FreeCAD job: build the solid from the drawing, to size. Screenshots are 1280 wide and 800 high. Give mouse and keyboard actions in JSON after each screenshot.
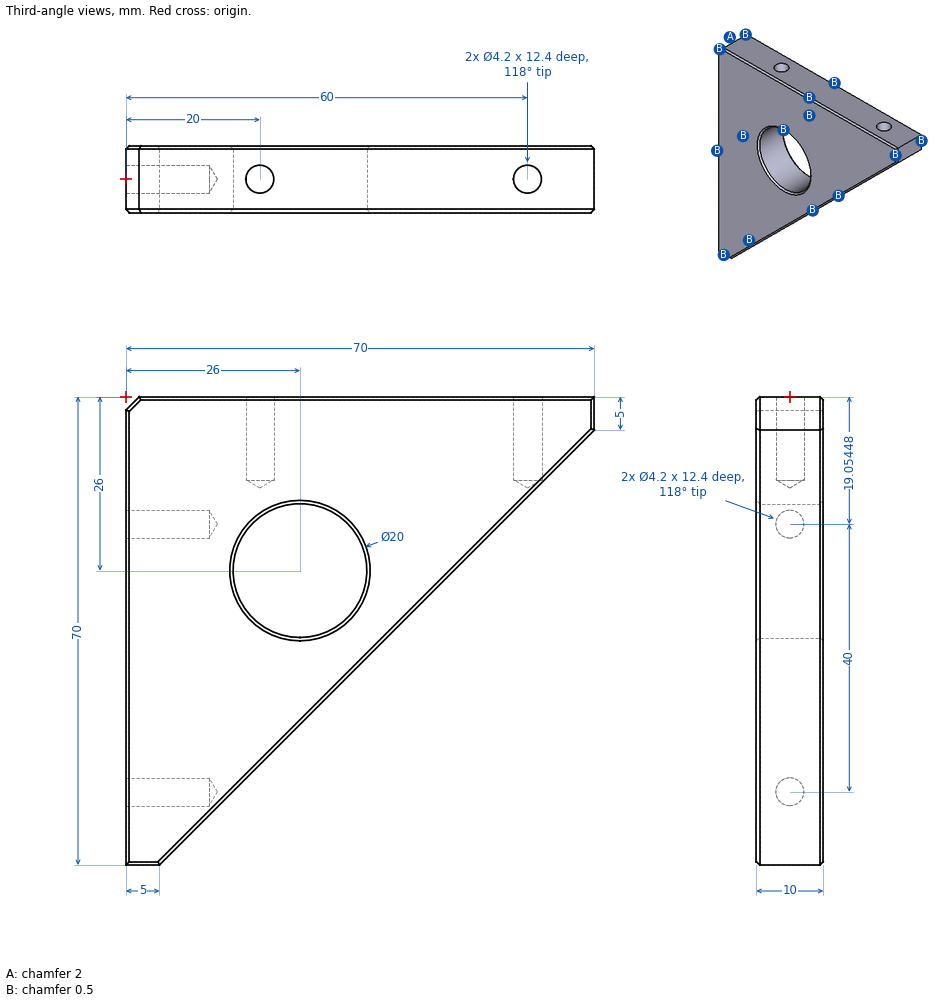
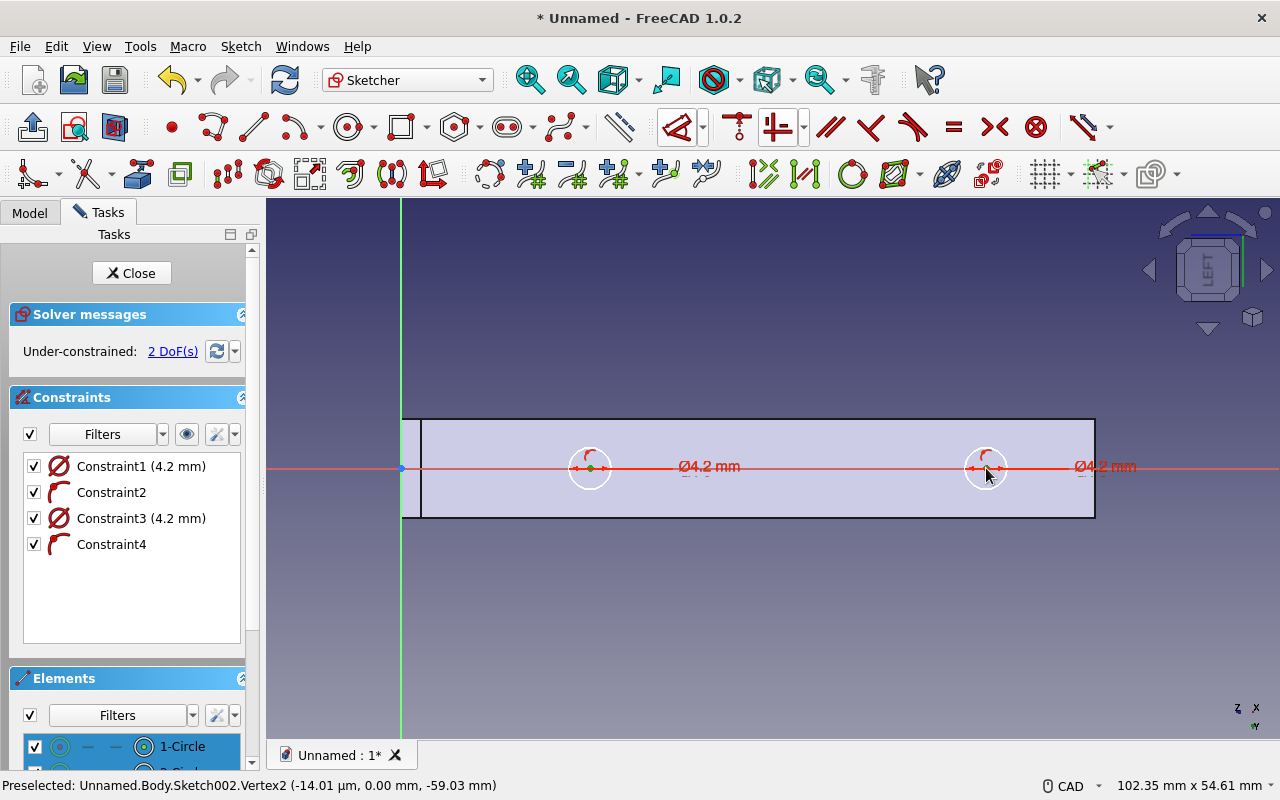
{"action": "key", "text": "l"}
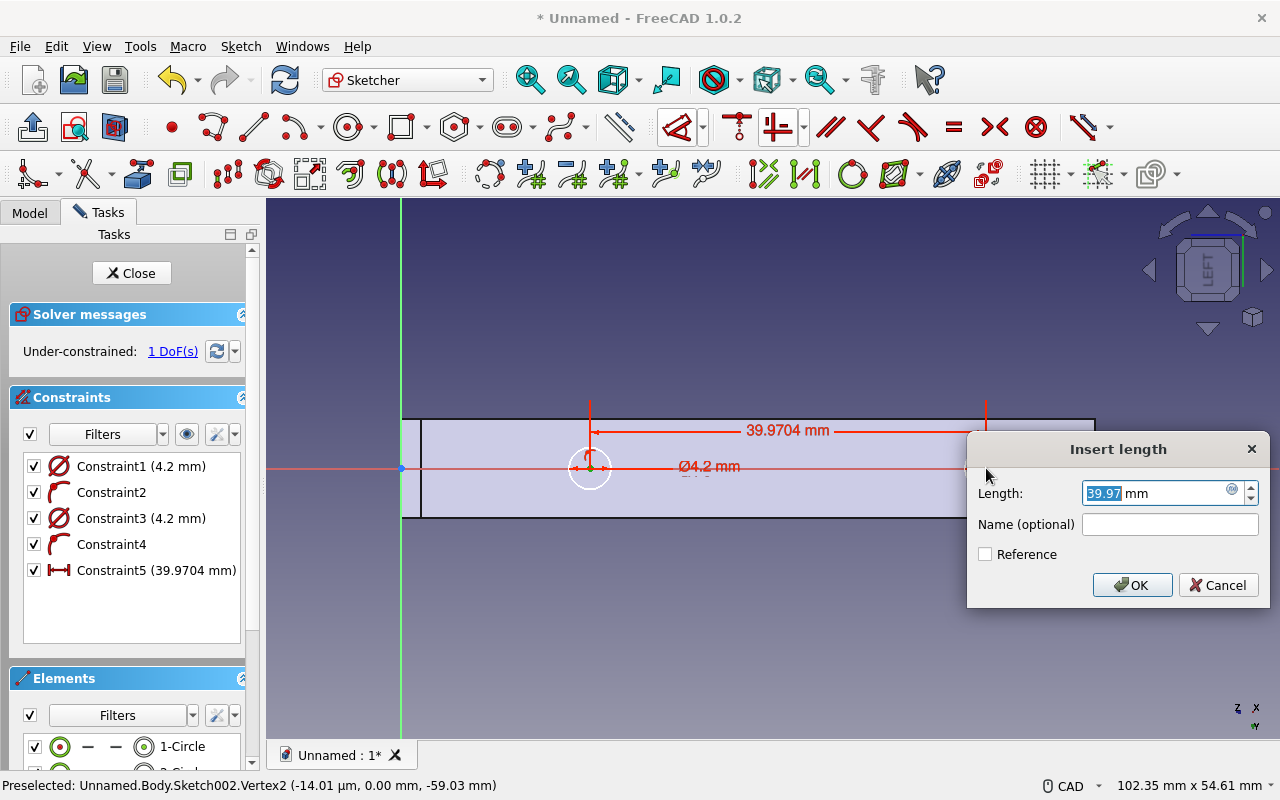
{"action": "type", "text": "40"}
{"action": "key", "text": "Return"}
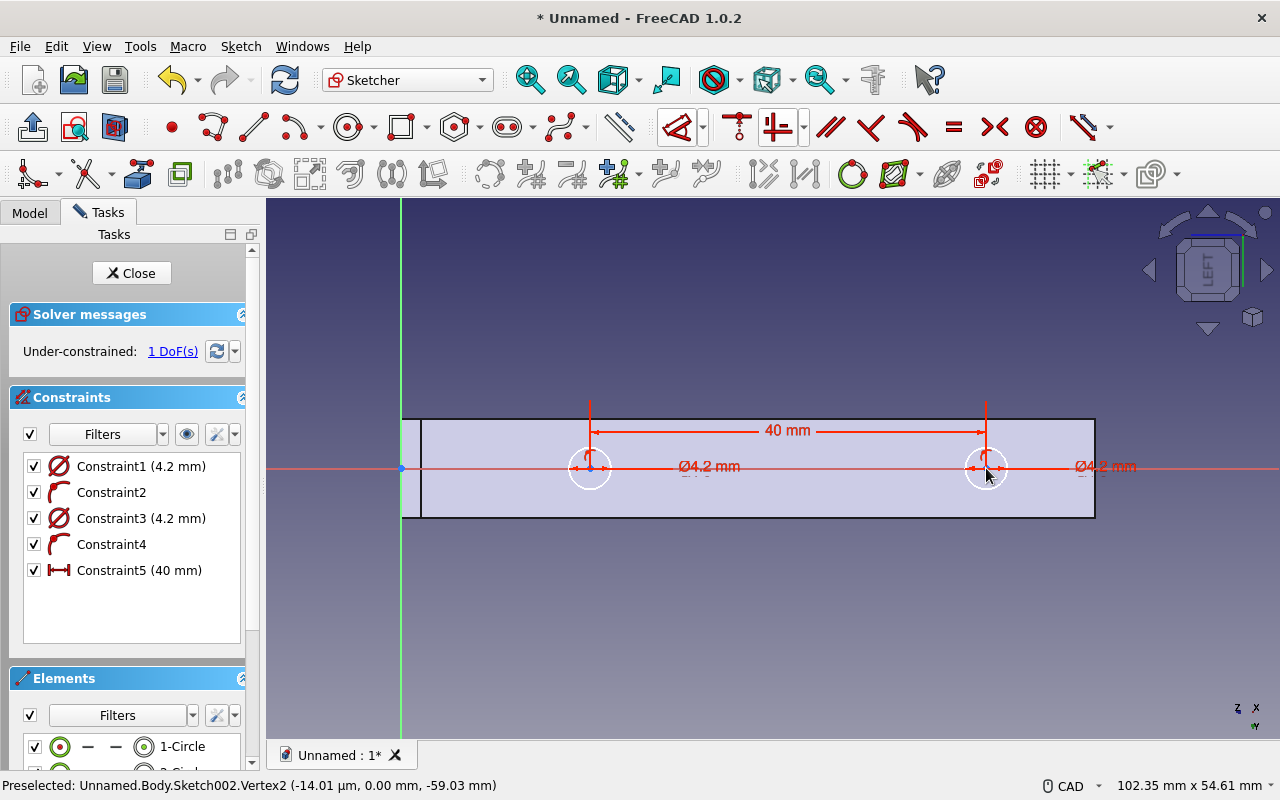
{"action": "left_click", "coordinate": [590, 468]}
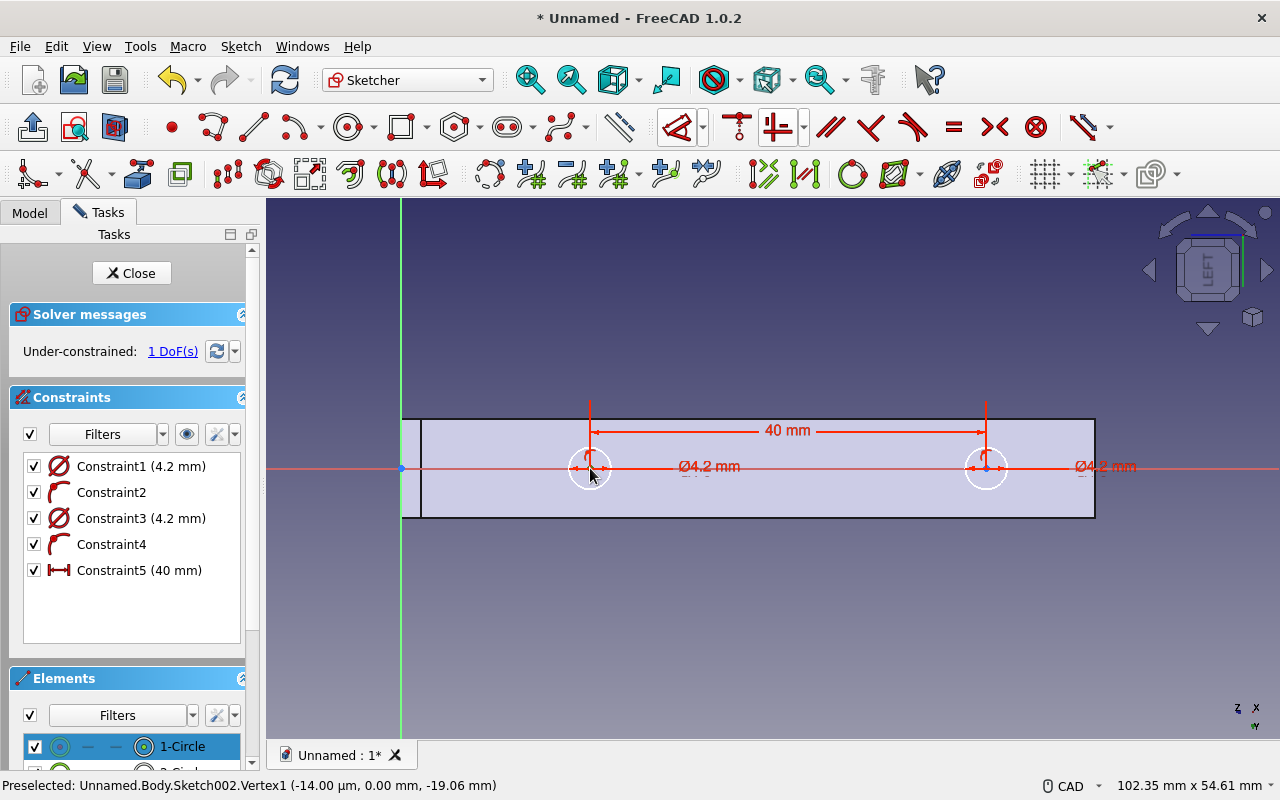
{"action": "left_click", "coordinate": [702, 128]}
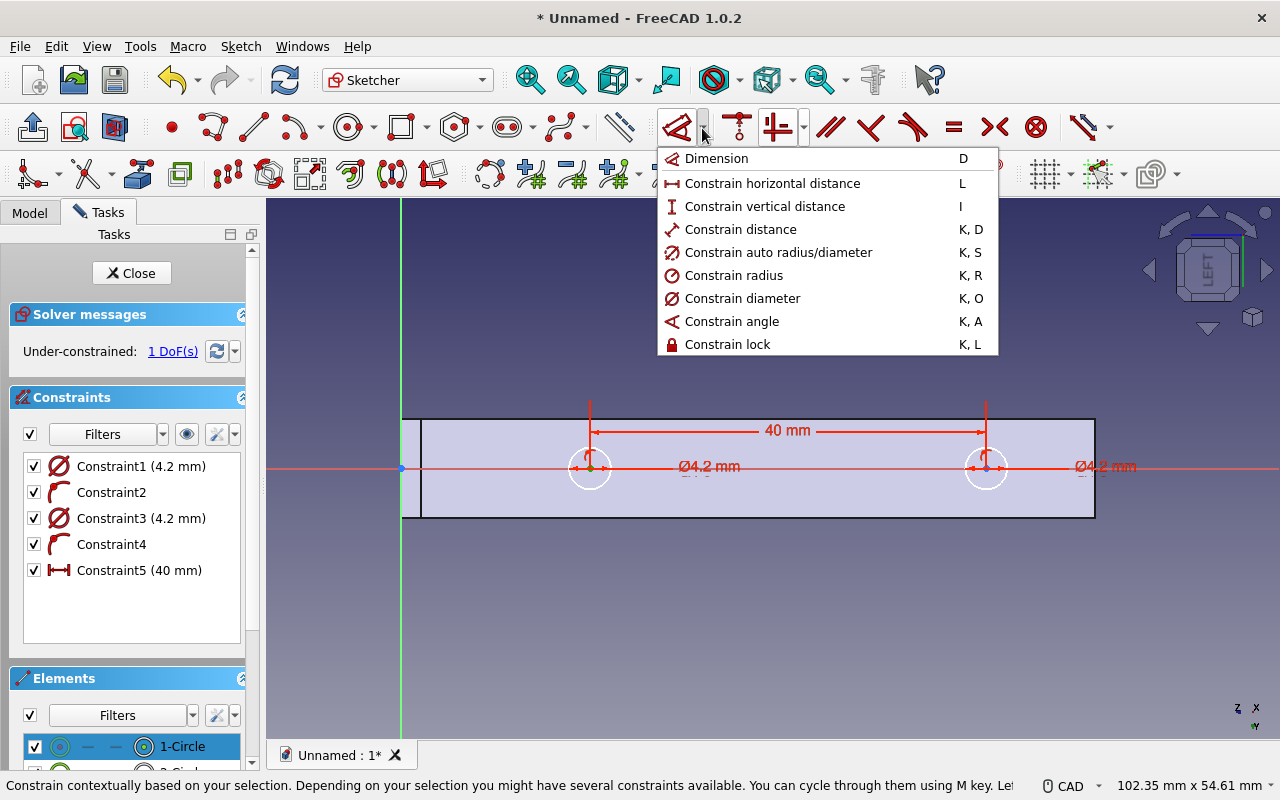
{"action": "left_click", "coordinate": [828, 184]}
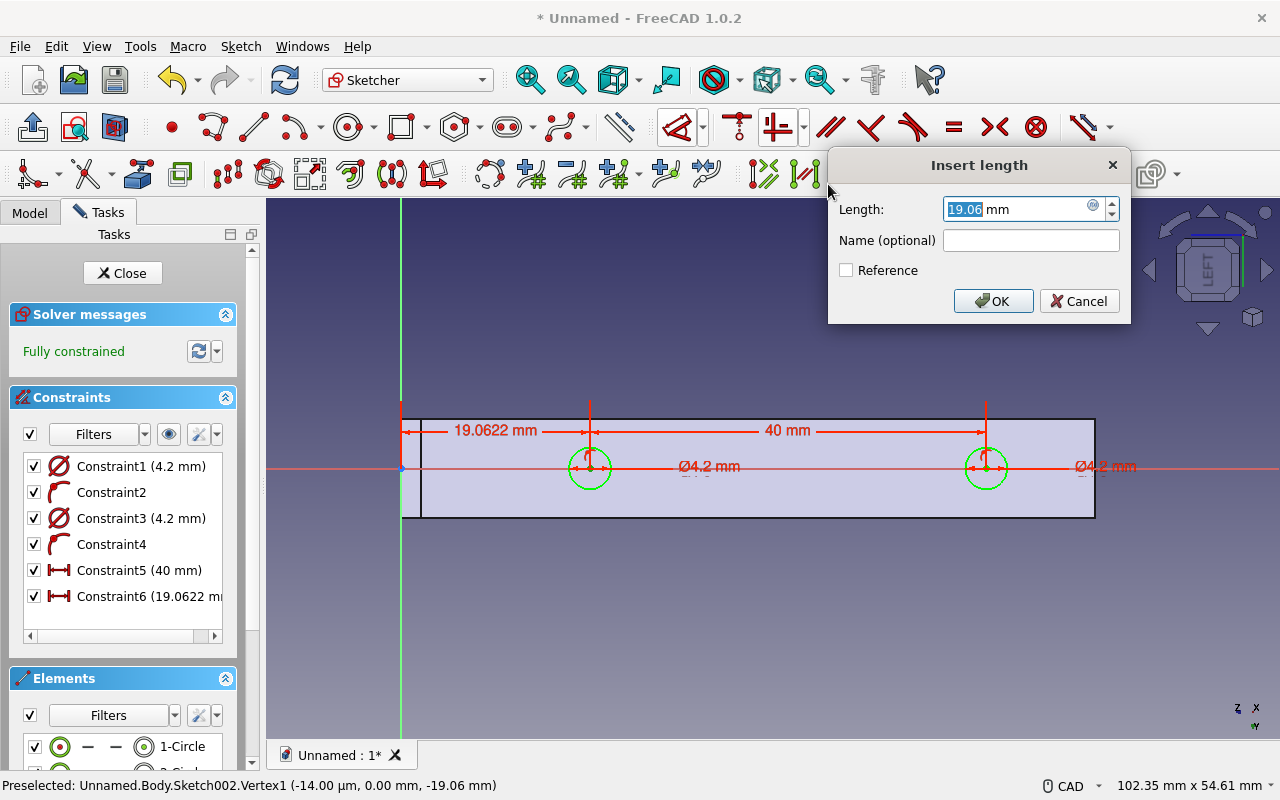
{"action": "type", "text": "19.05448"}
{"action": "key", "text": "Return"}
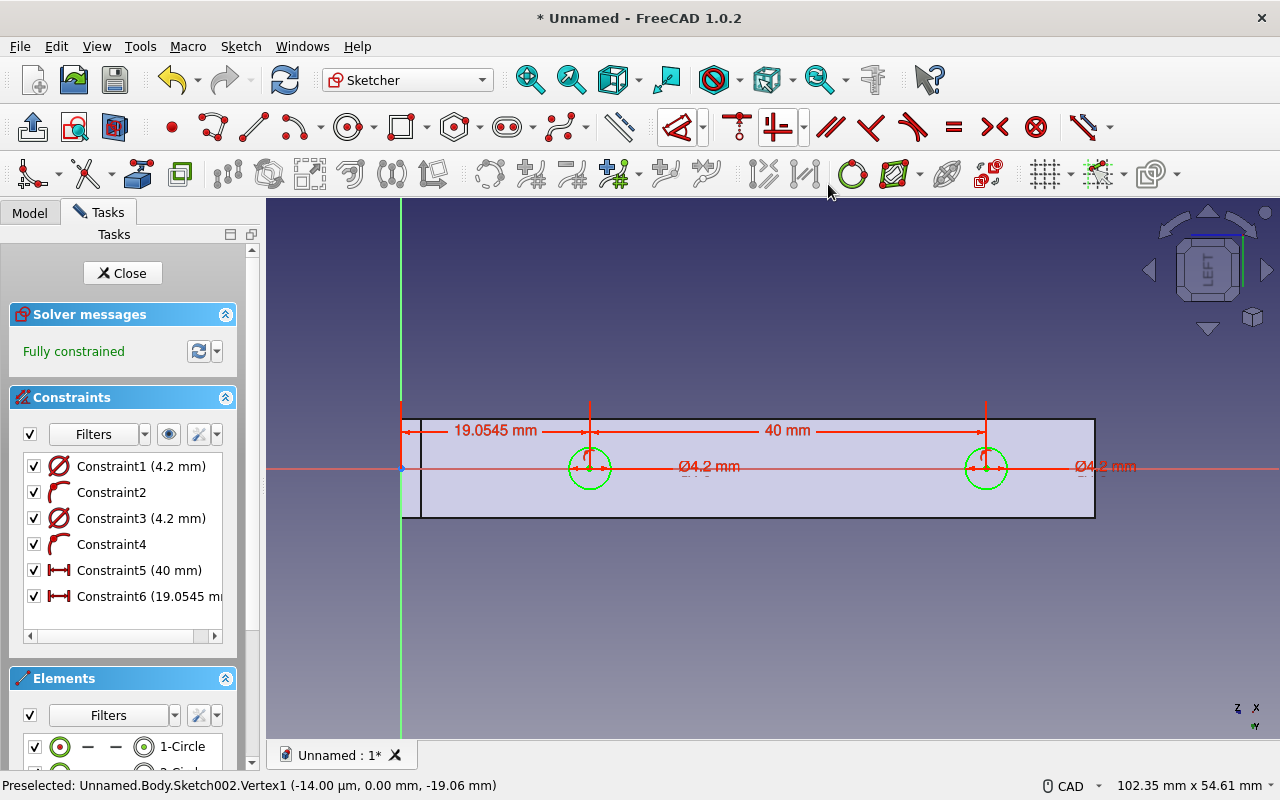
{"action": "left_click", "coordinate": [123, 273]}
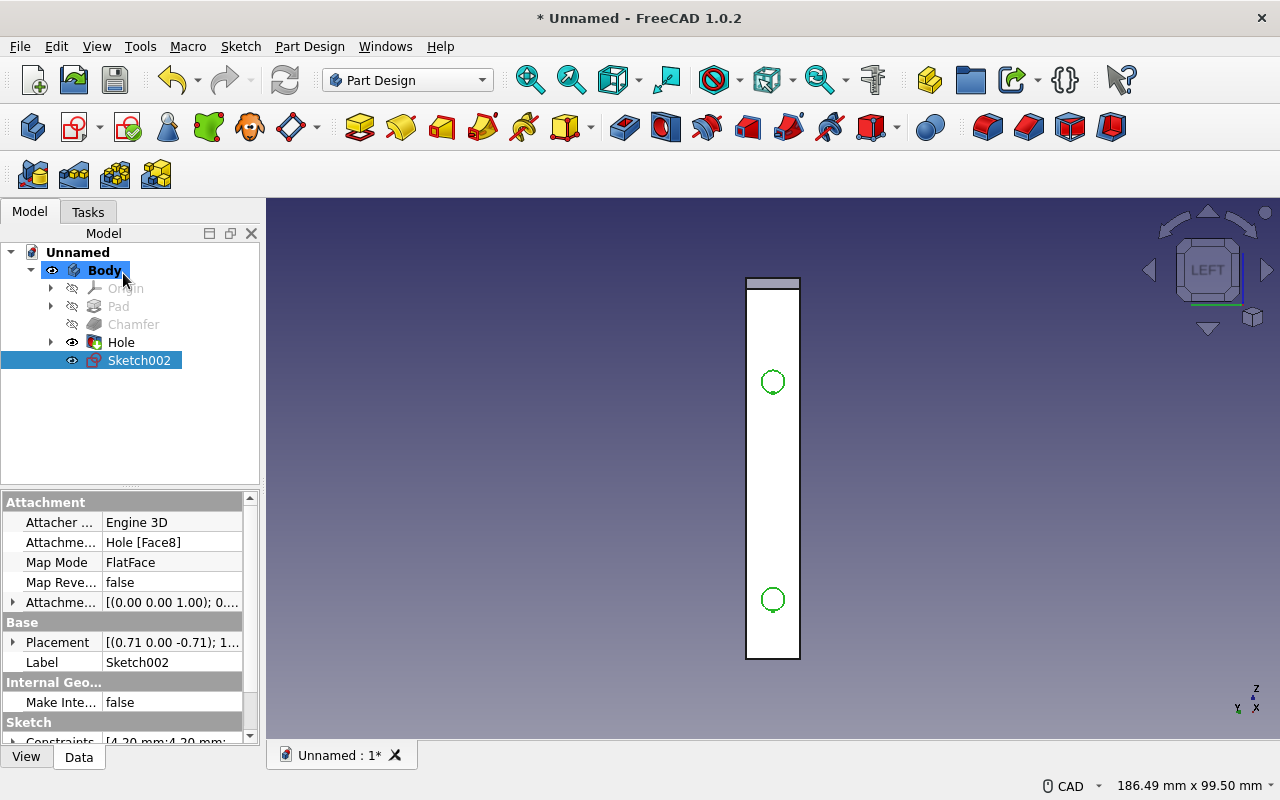
{"action": "left_click", "coordinate": [666, 128]}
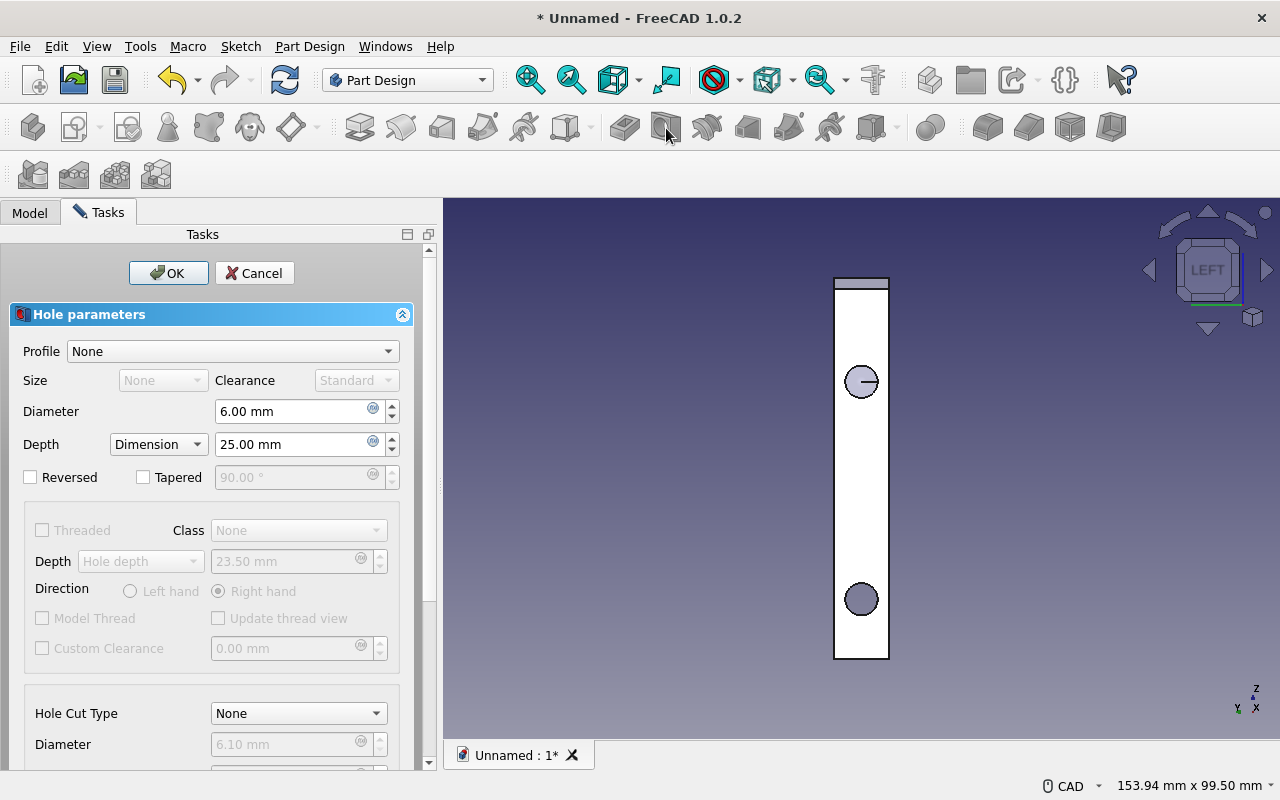
{"action": "triple_click", "coordinate": [300, 412]}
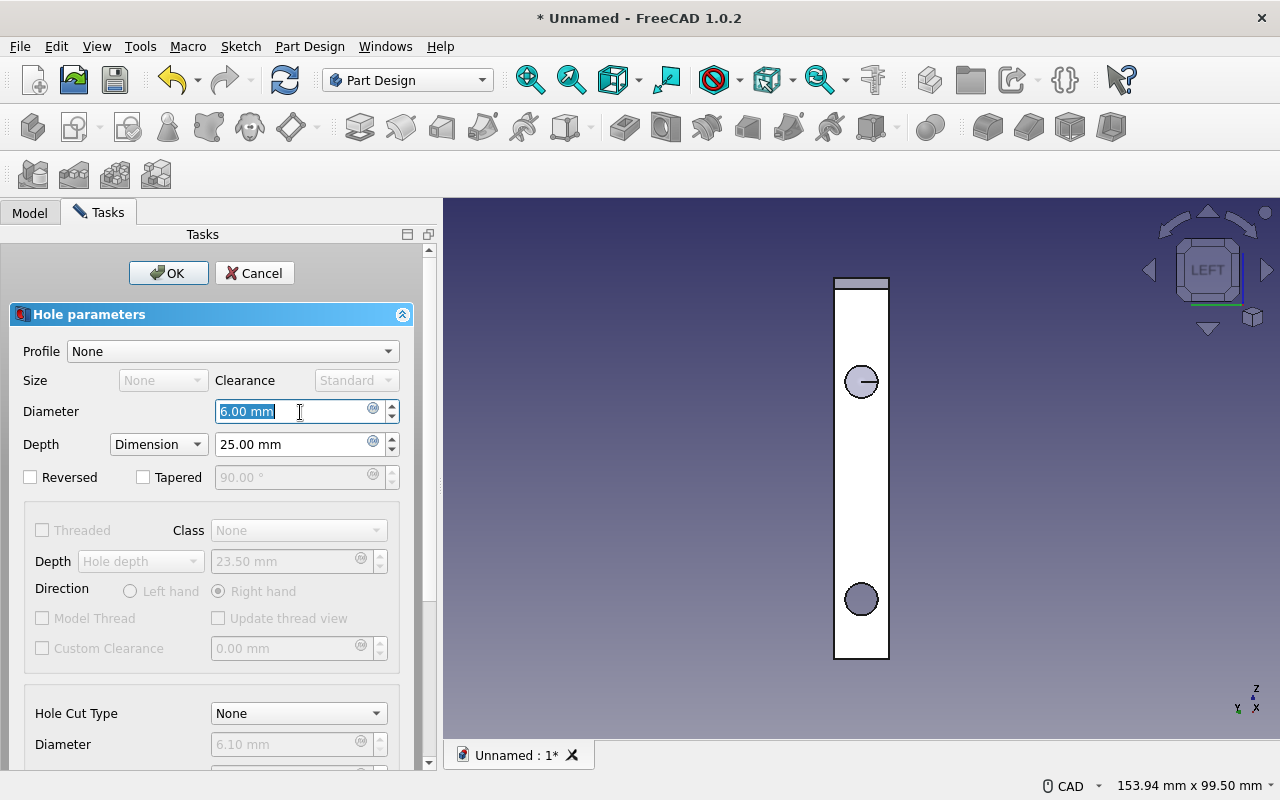
{"action": "type", "text": "4.2"}
{"action": "key", "text": "Tab"}